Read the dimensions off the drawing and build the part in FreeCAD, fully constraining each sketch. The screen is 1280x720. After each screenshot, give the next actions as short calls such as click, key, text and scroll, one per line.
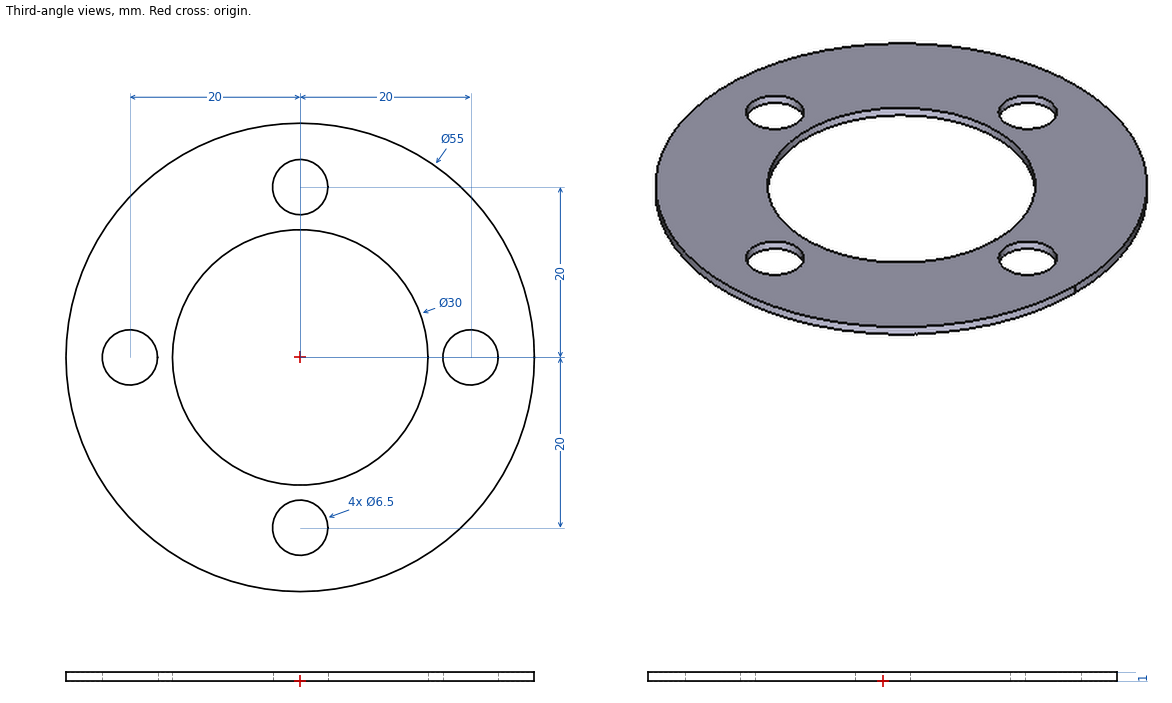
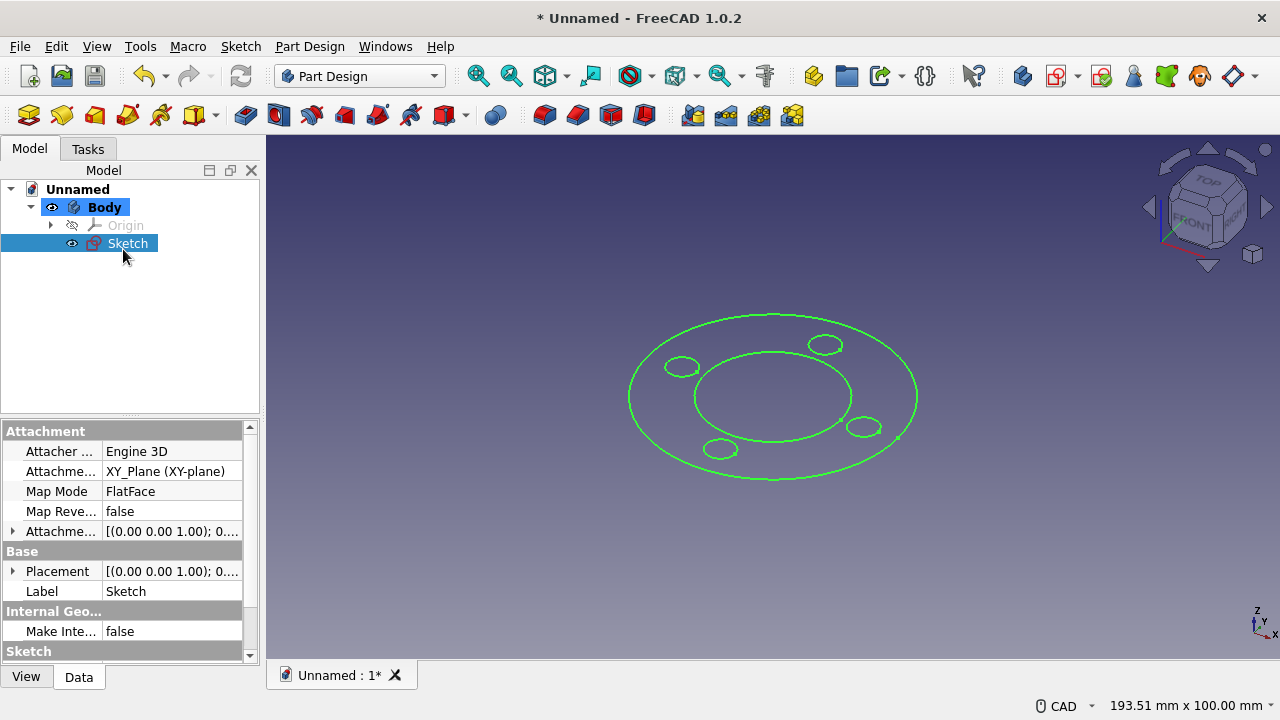
click(29, 116)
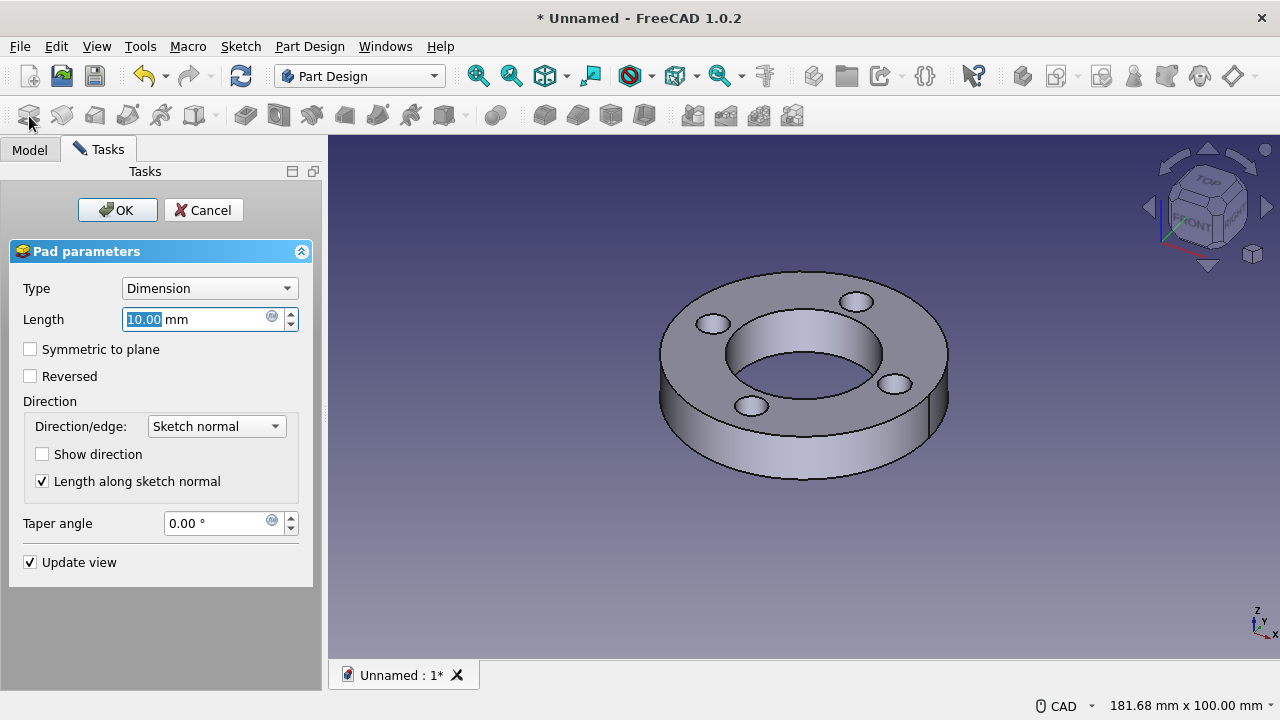
text(1)
key(Tab)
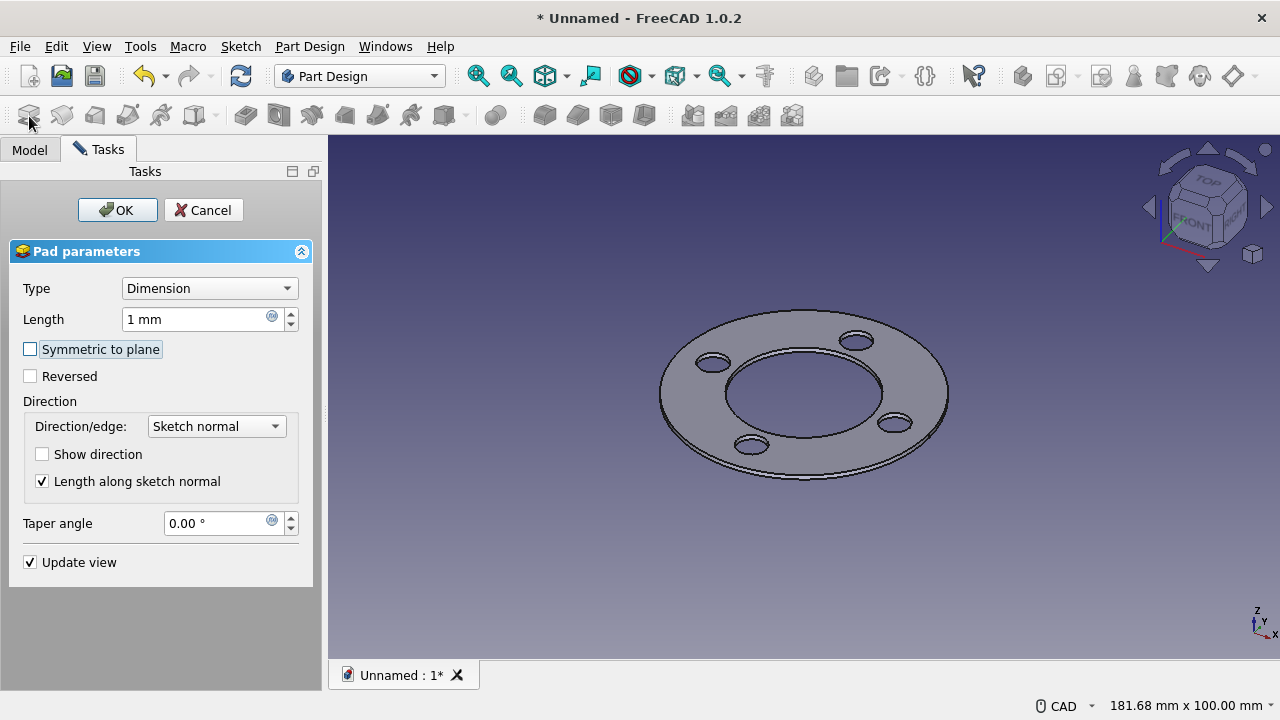
click(118, 210)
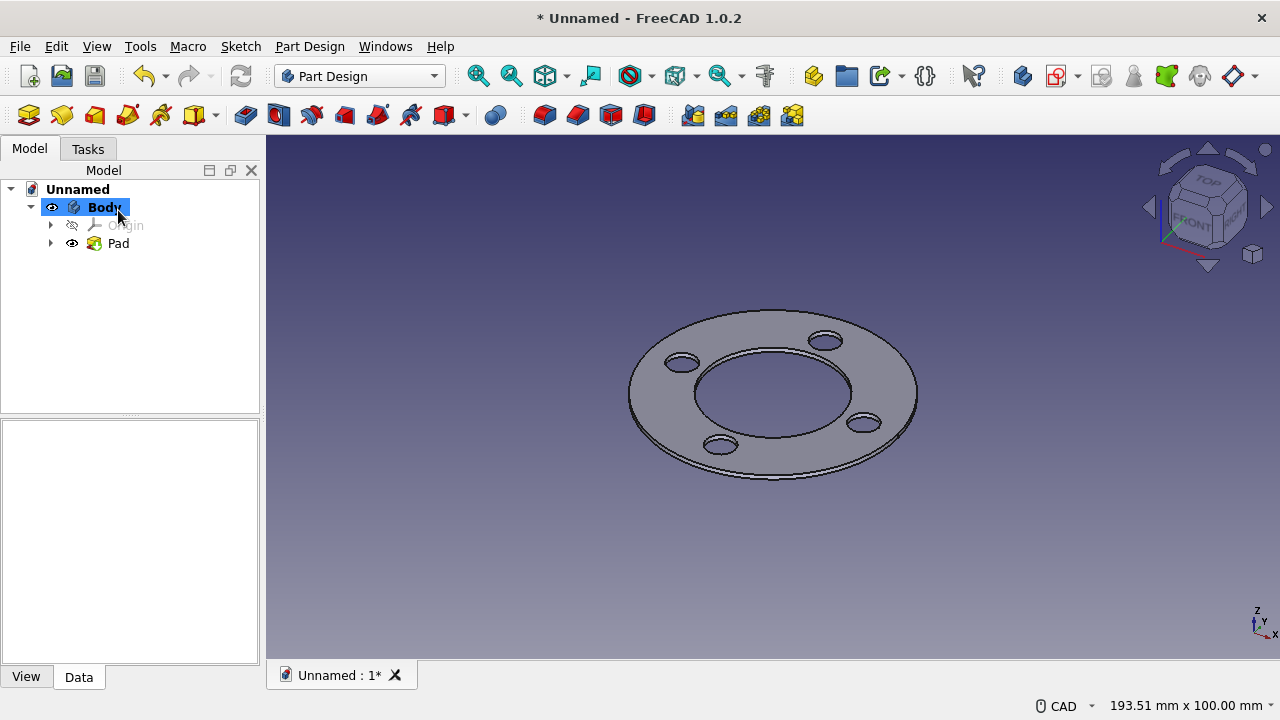
key(0)